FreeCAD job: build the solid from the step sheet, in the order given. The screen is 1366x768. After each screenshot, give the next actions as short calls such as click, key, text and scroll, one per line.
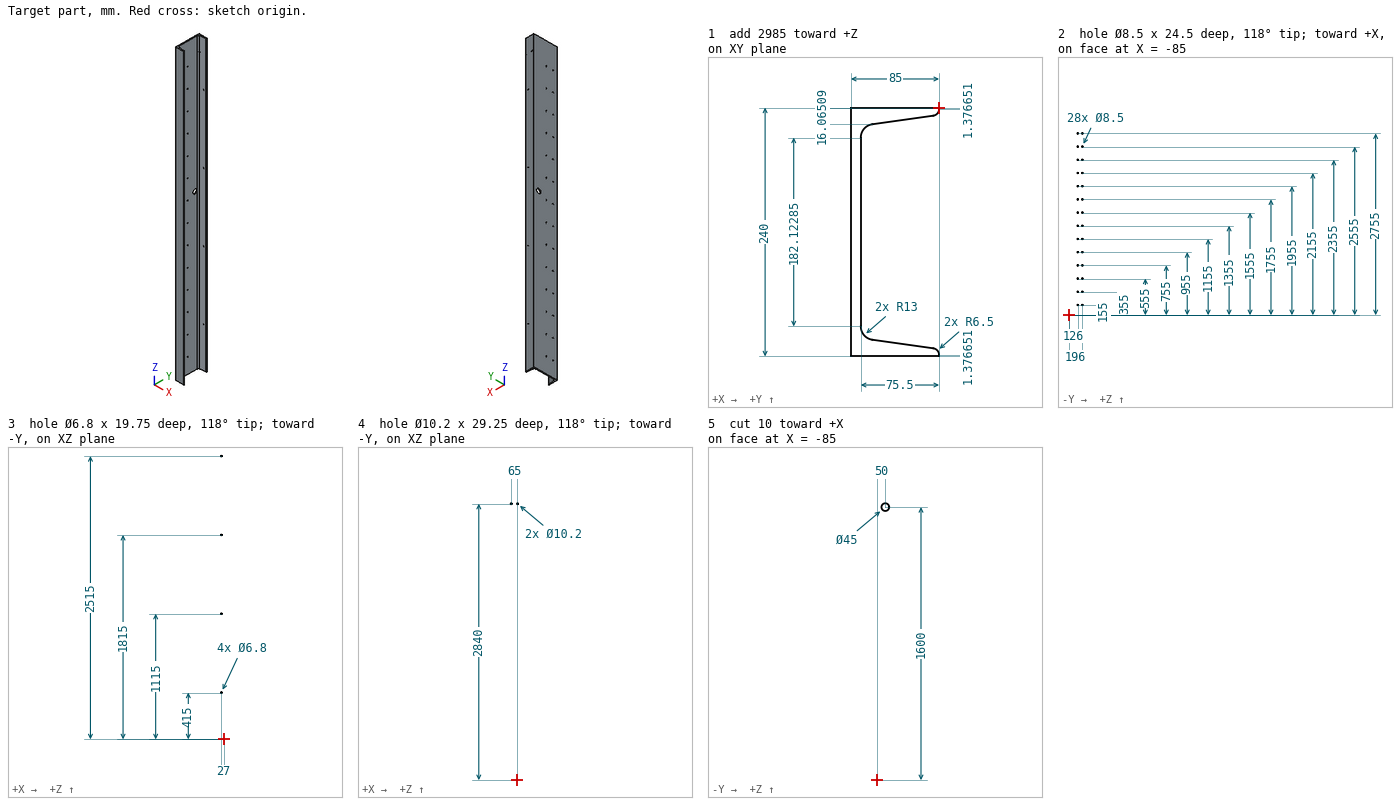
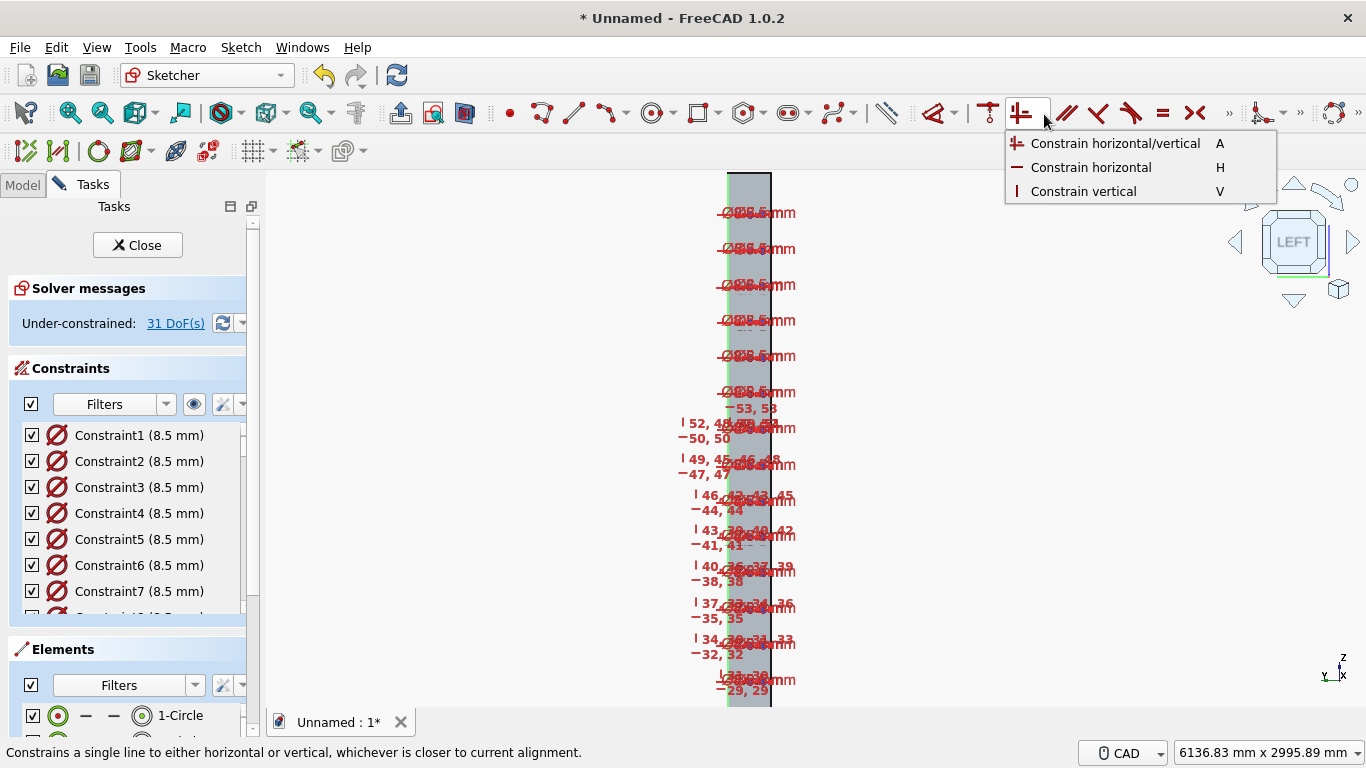
click(1141, 191)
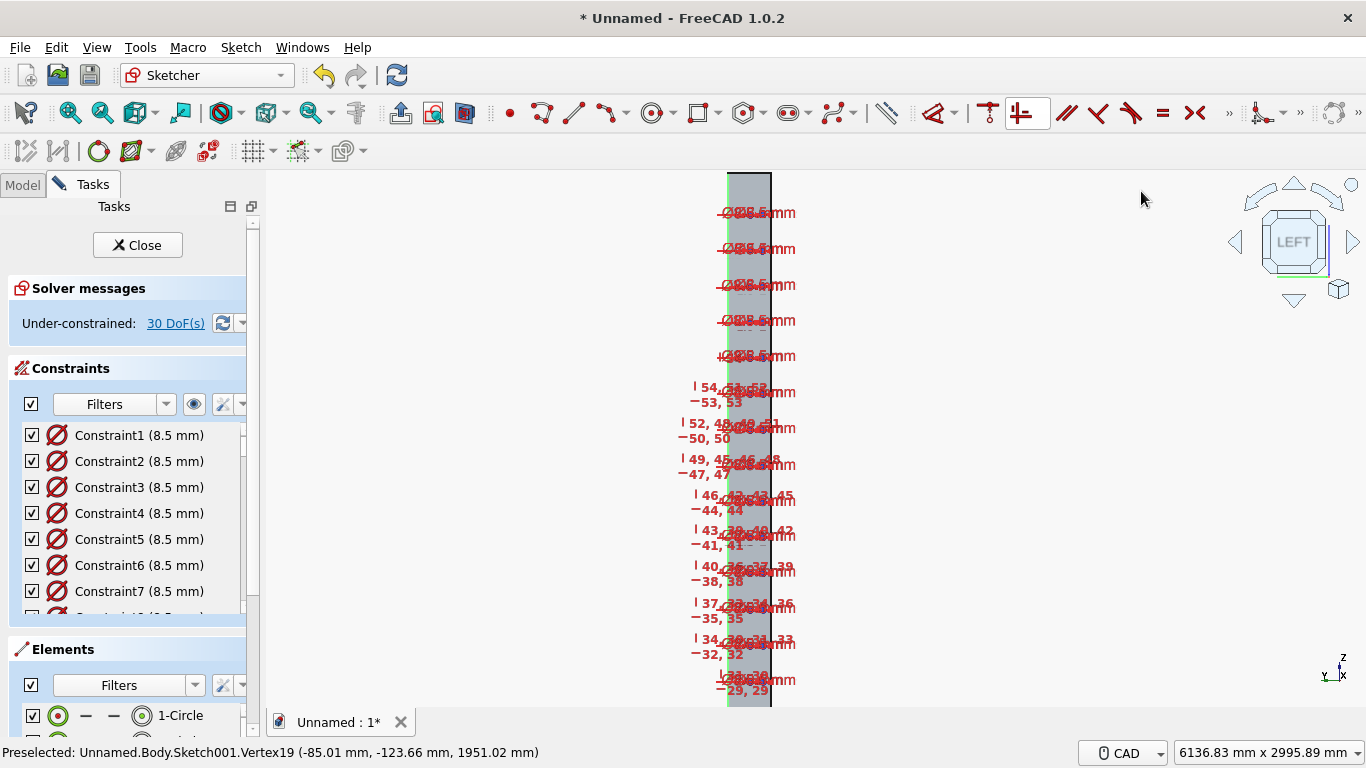
click(763, 394)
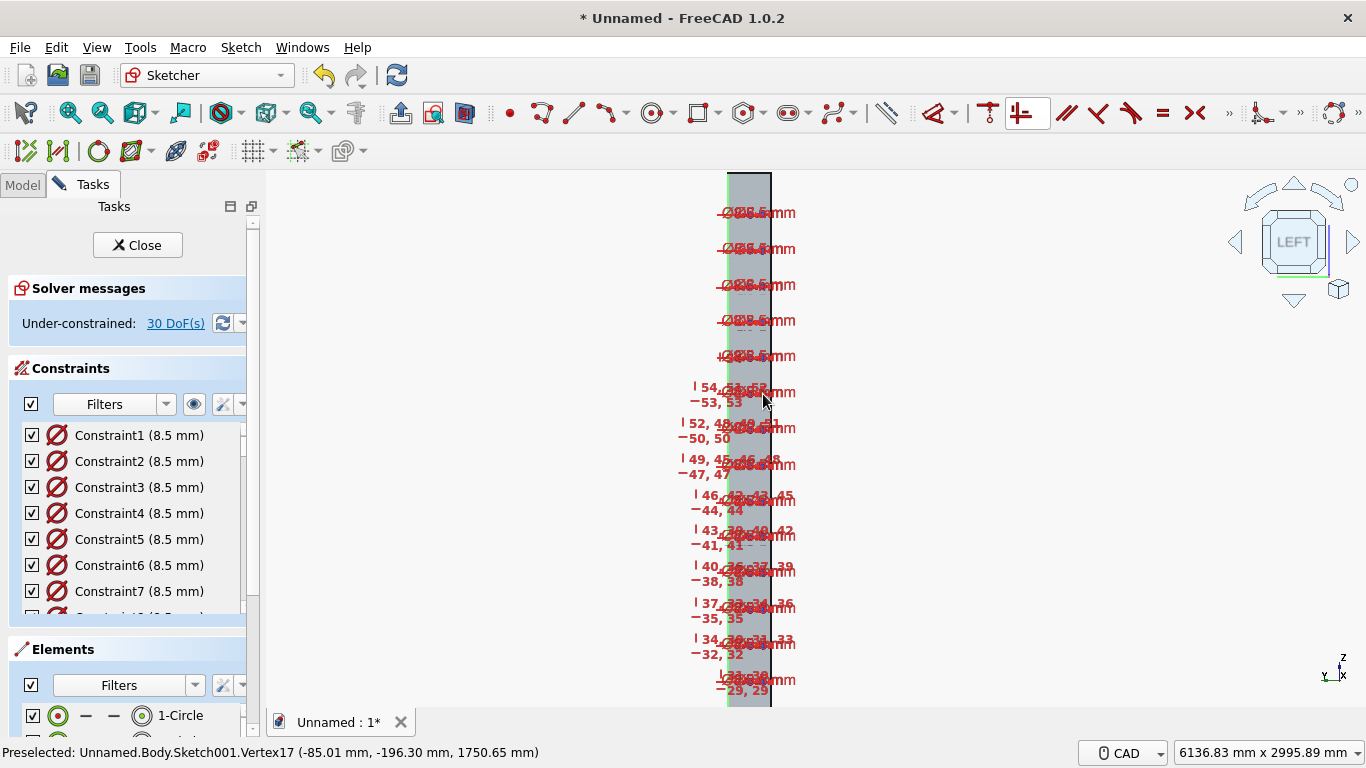
click(763, 358)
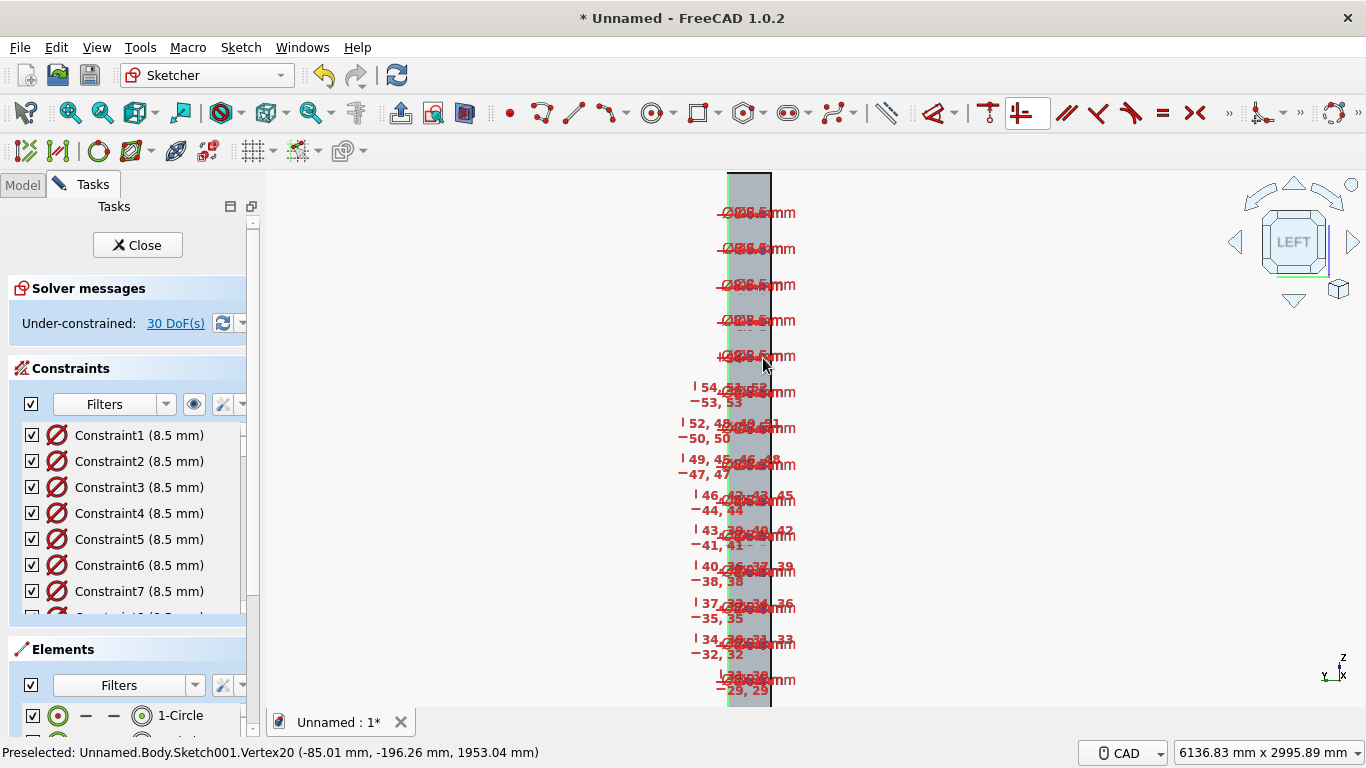
key(v)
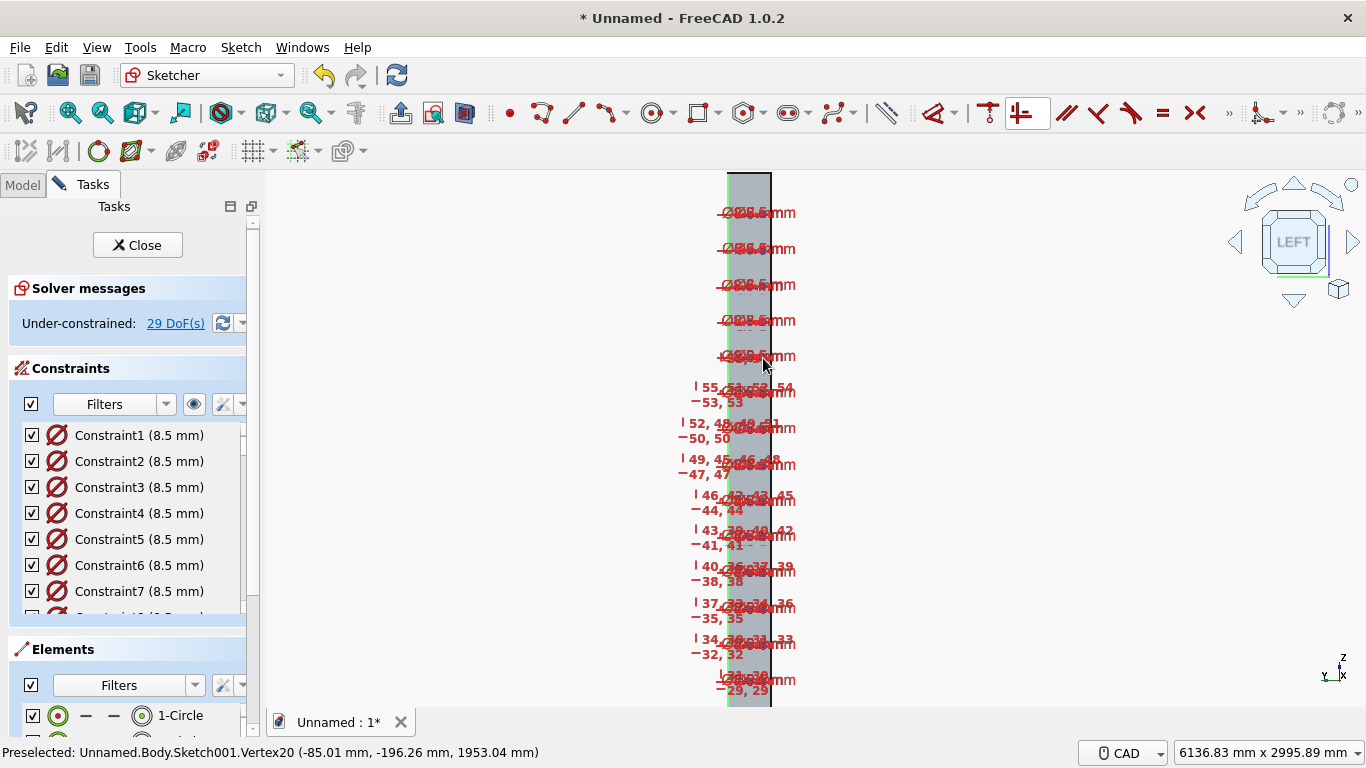
scroll(750, 358, up, 4)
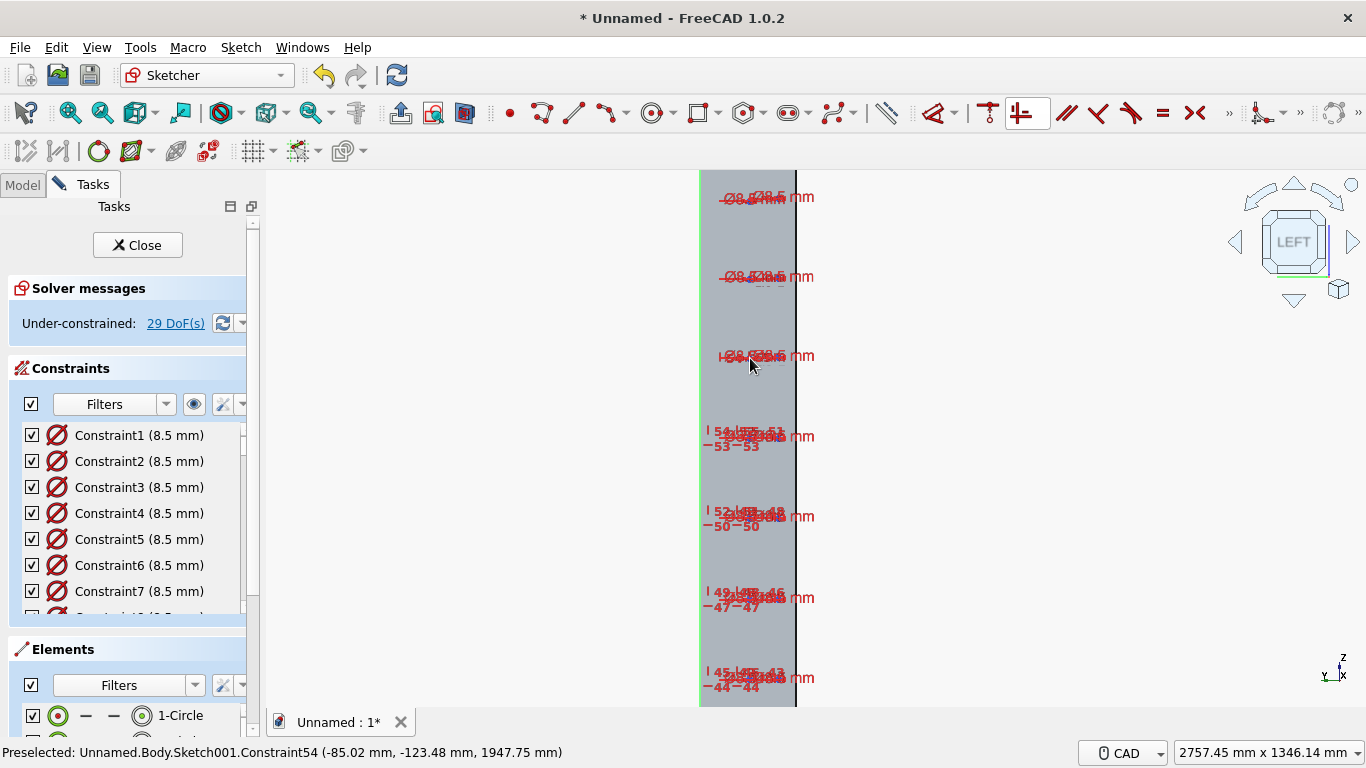
scroll(750, 358, up, 4)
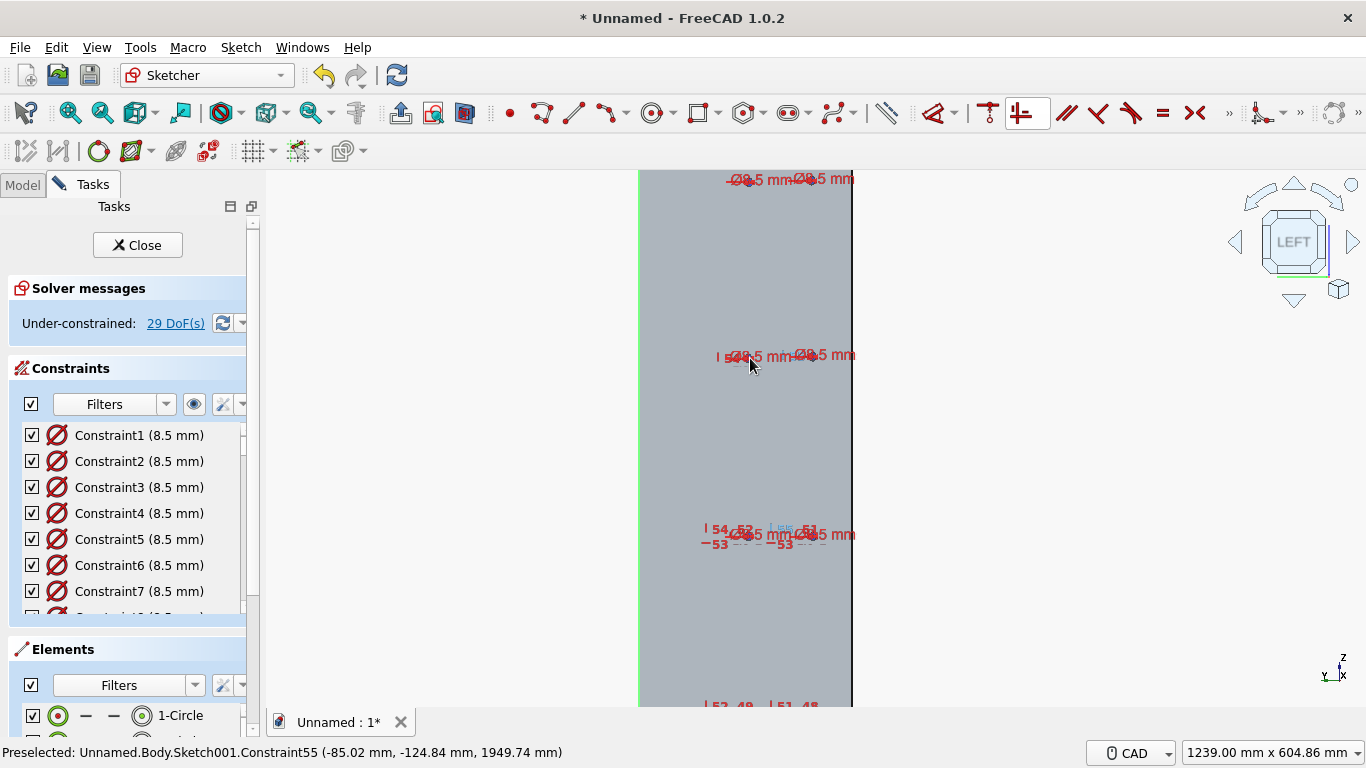
click(748, 359)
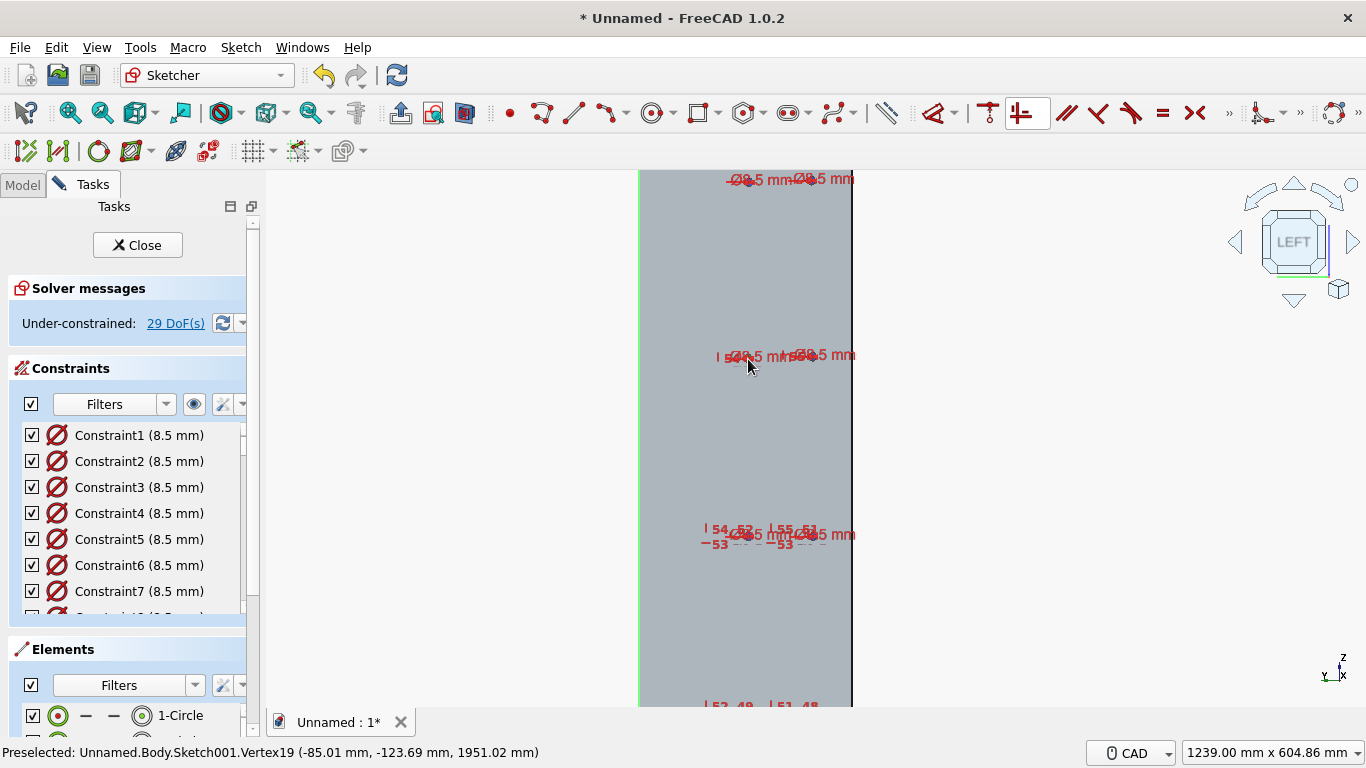
scroll(751, 372, down, 10)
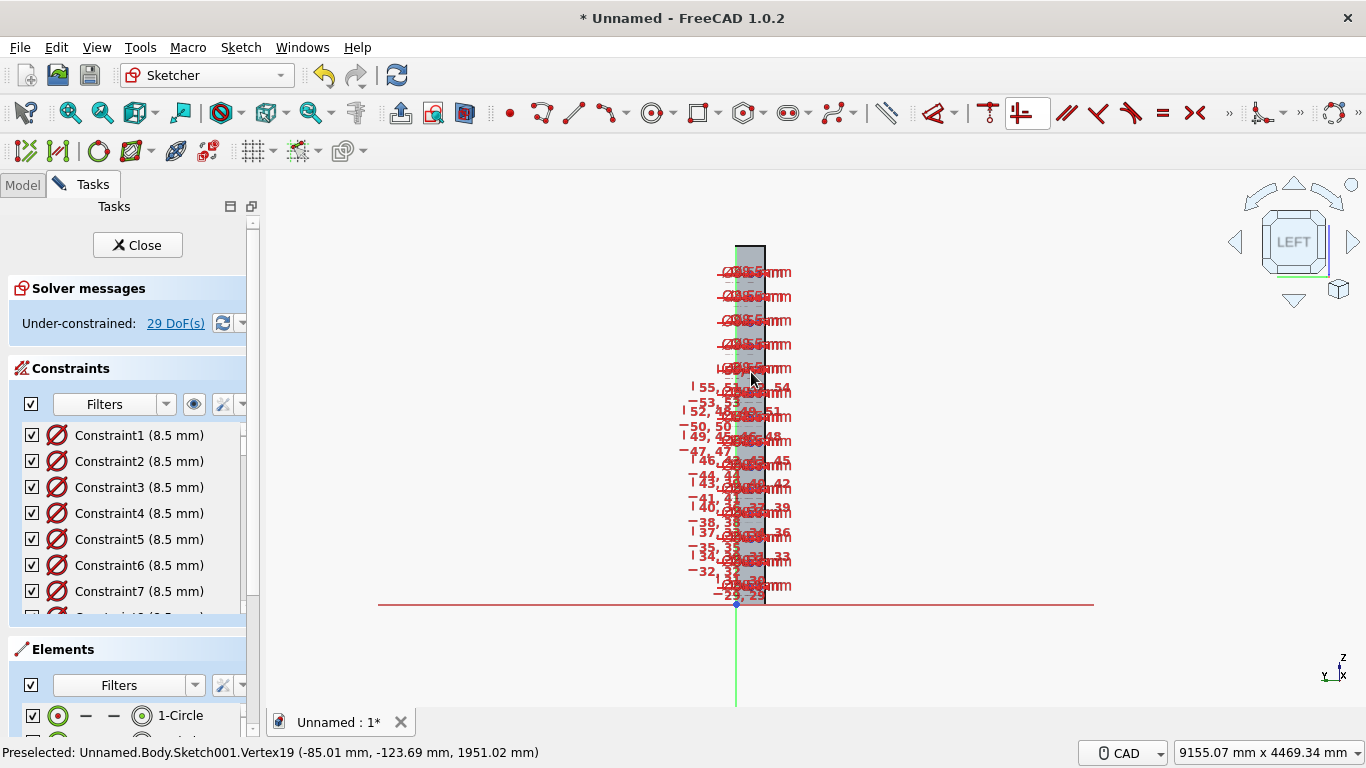
scroll(760, 370, up, 2)